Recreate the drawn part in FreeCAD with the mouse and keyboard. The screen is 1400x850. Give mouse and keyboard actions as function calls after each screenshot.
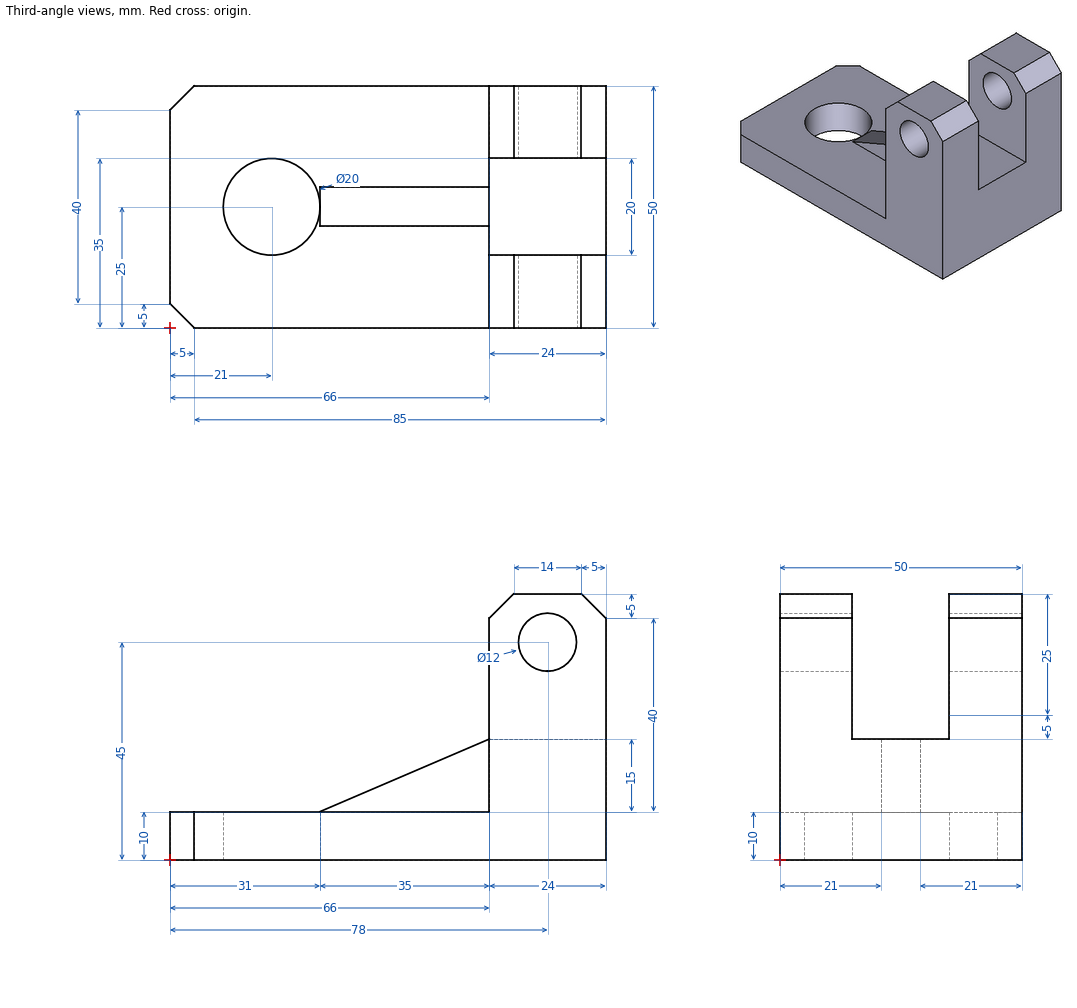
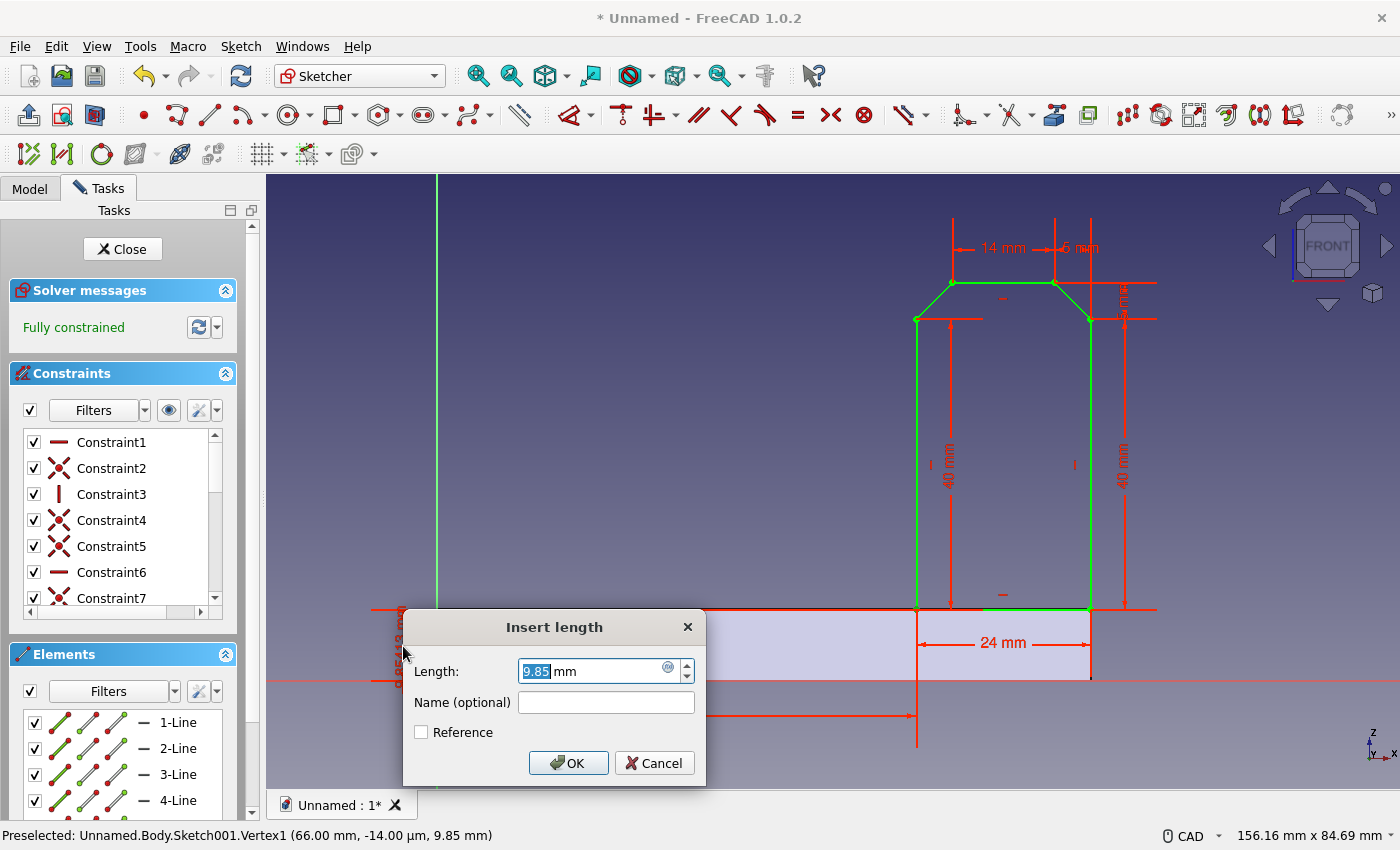
text(10)
key(Return)
key(Escape)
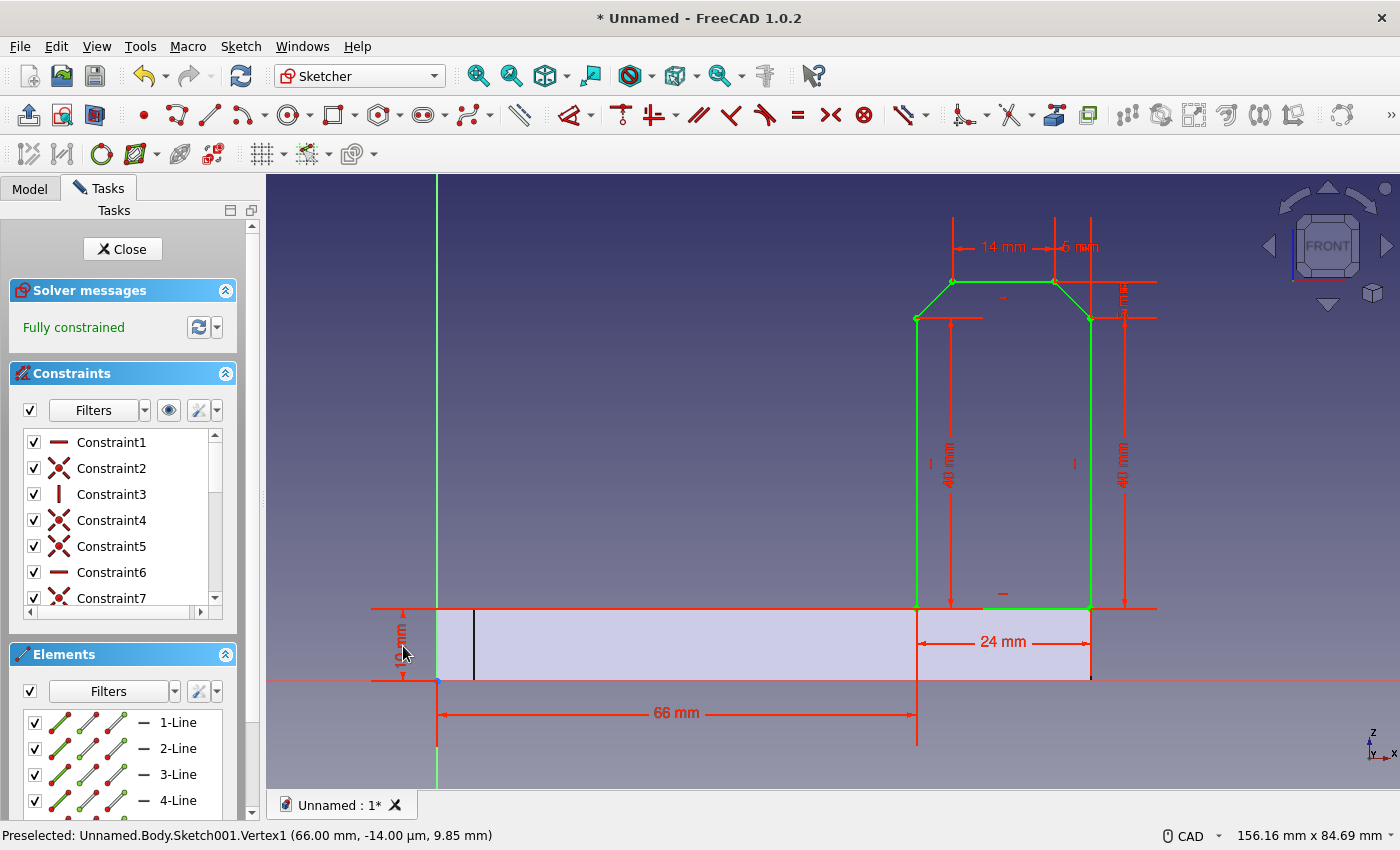
click(123, 249)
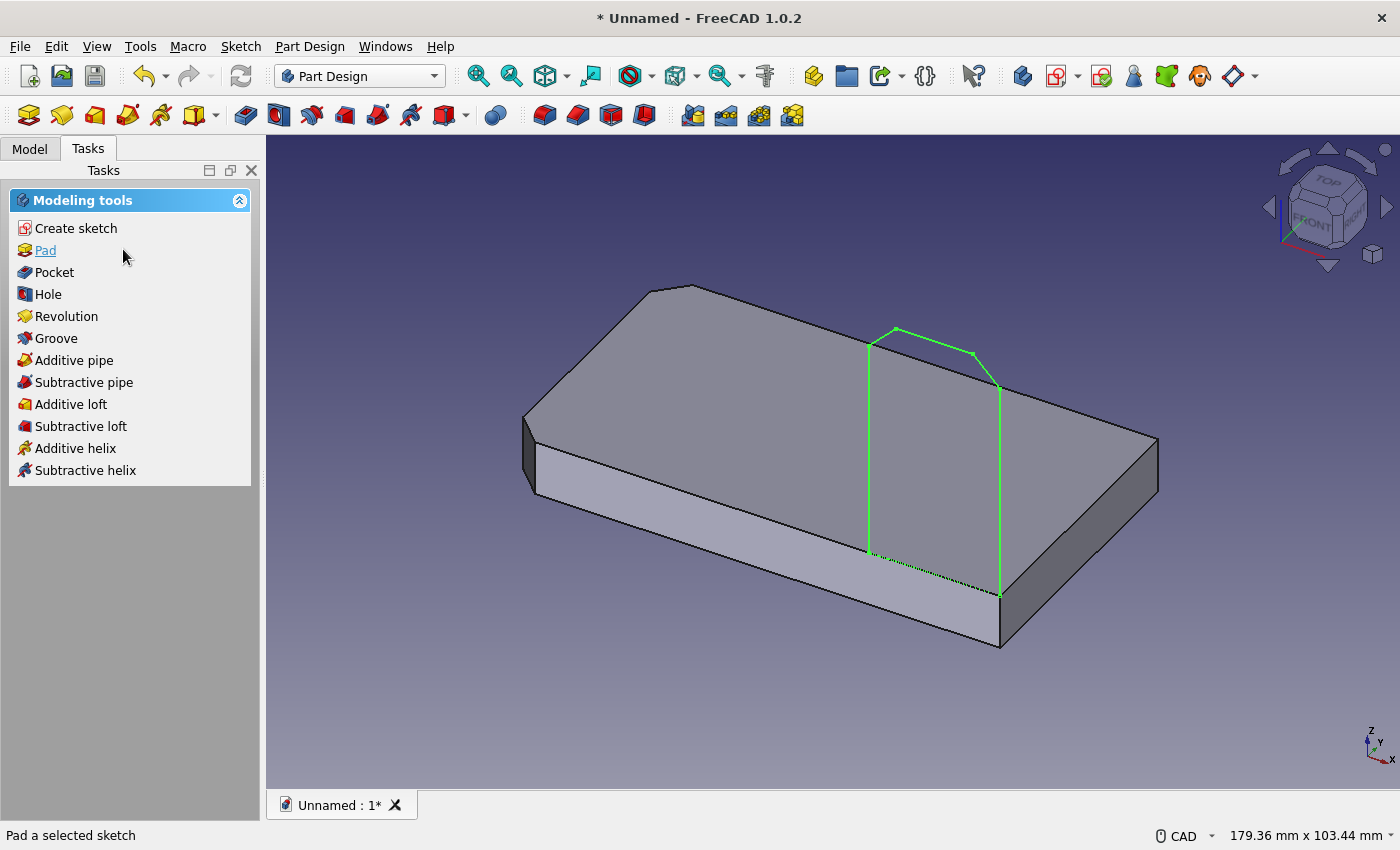
click(29, 116)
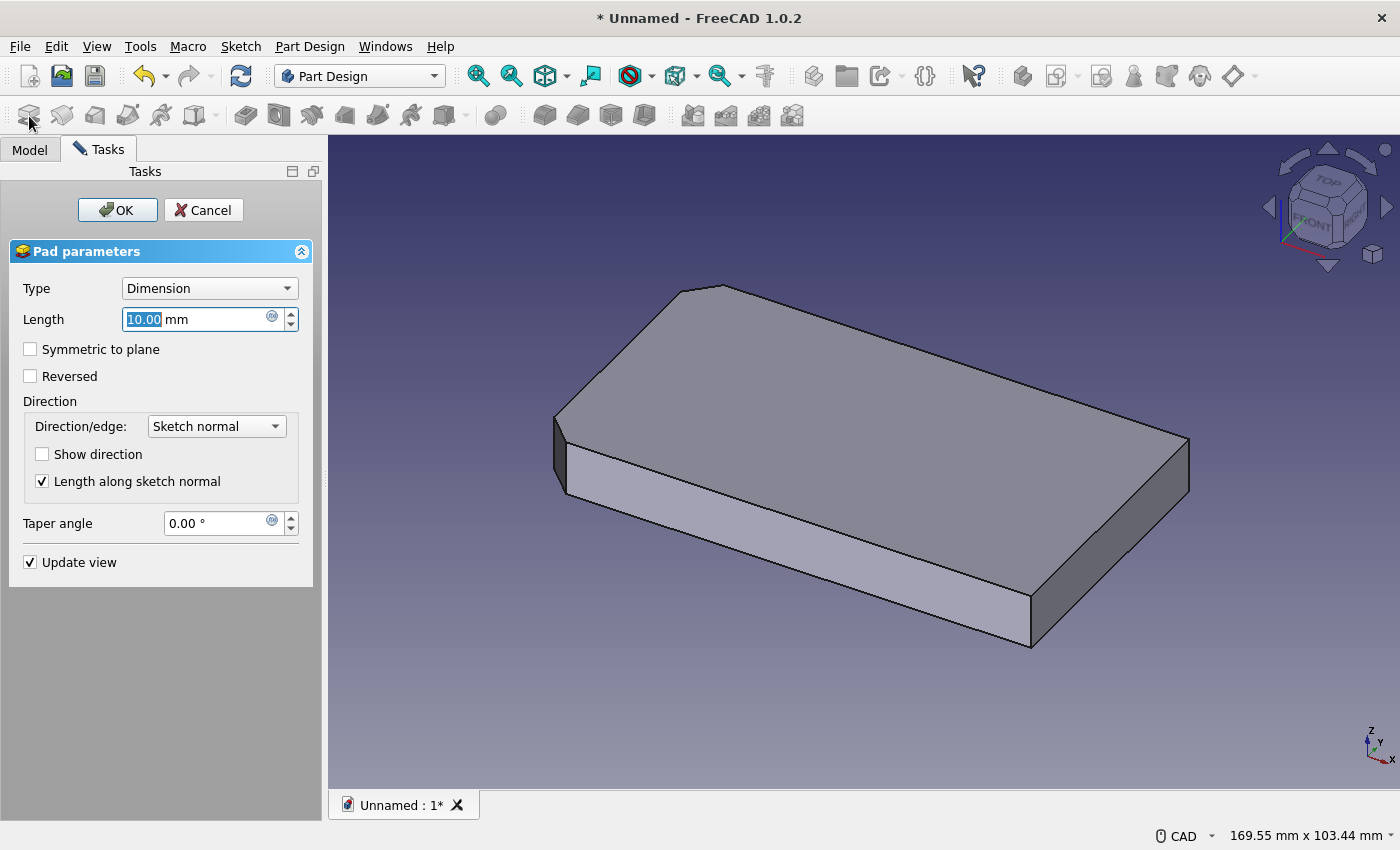
text(50)
key(Tab)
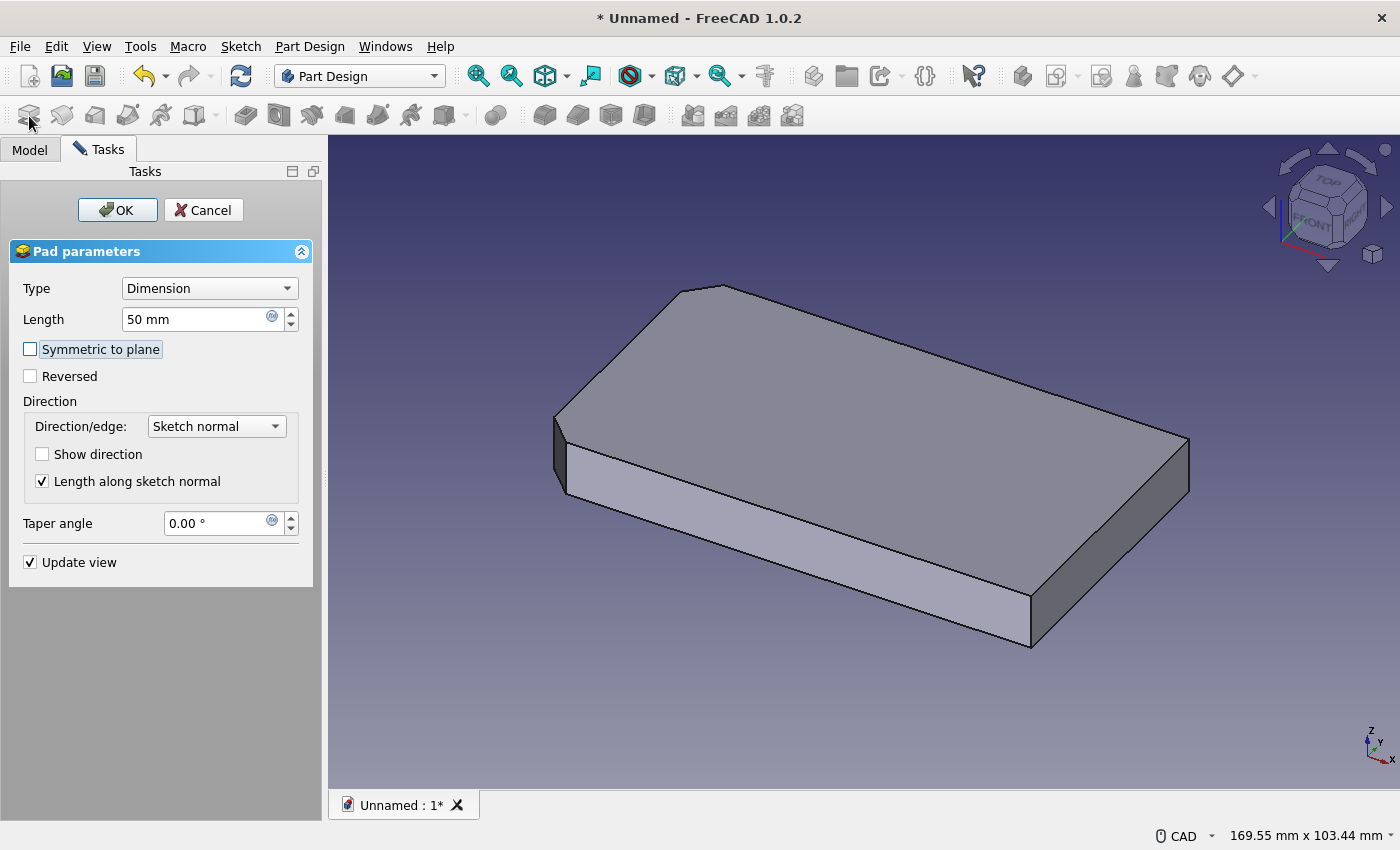
click(31, 376)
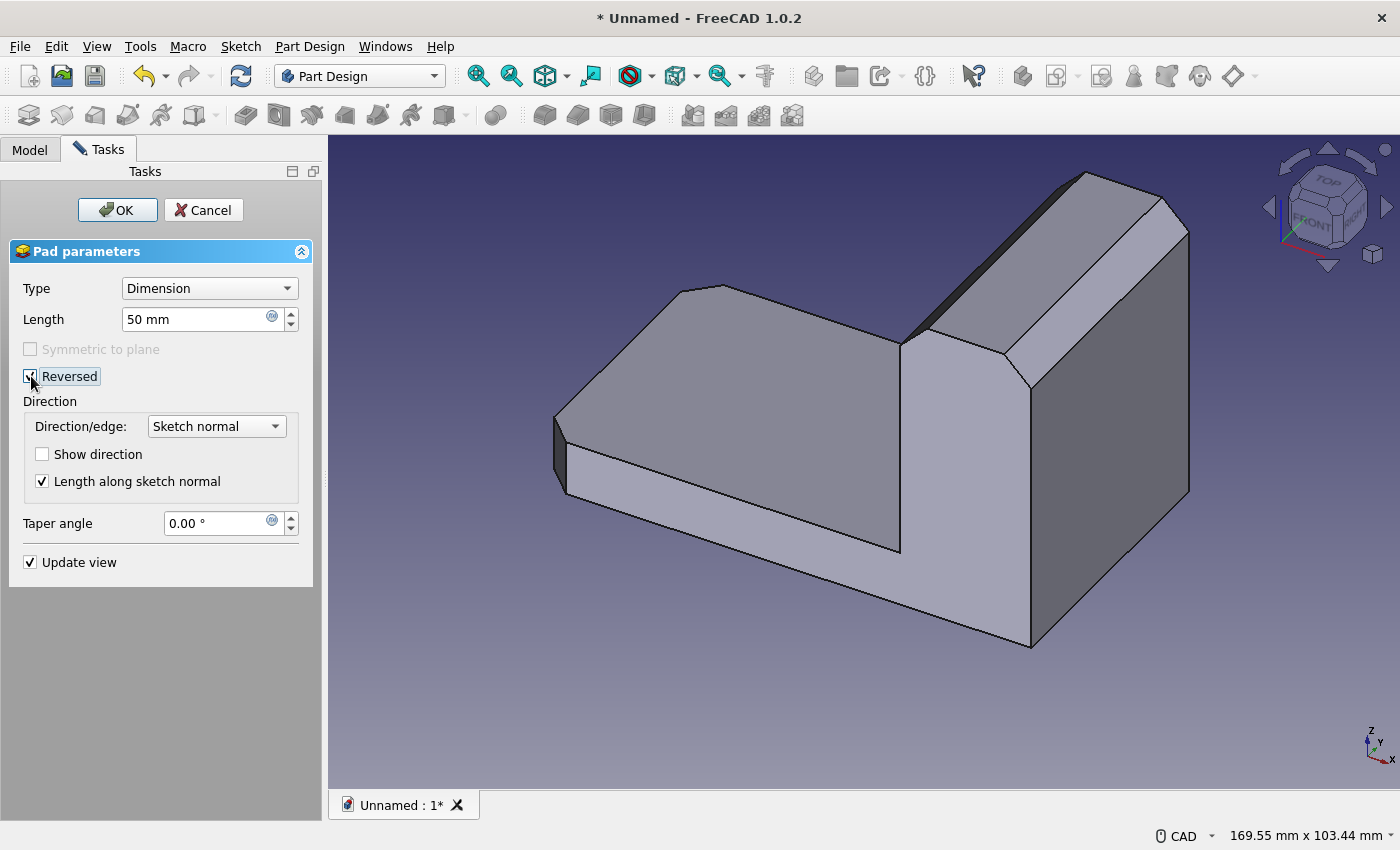
click(118, 210)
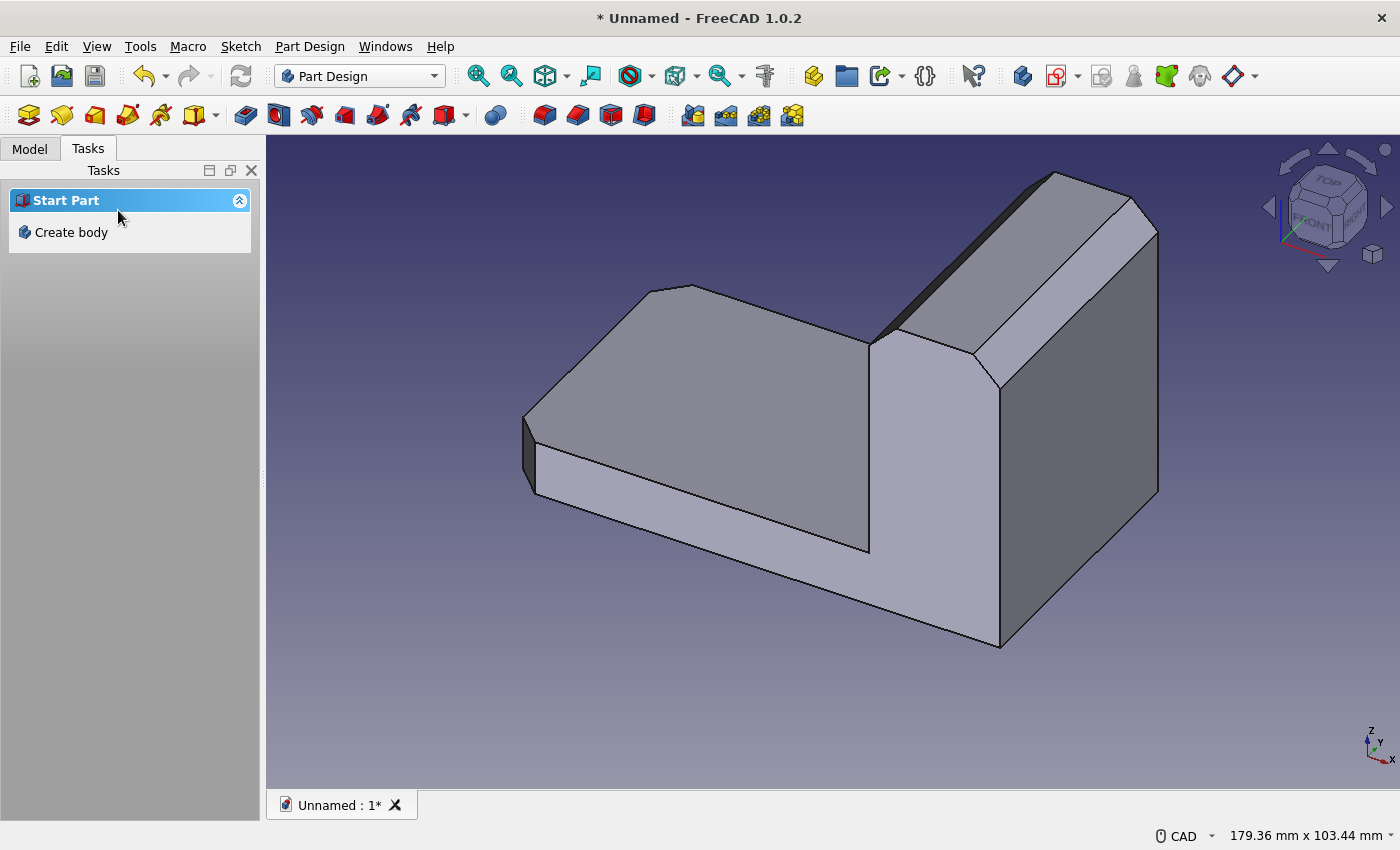
click(479, 76)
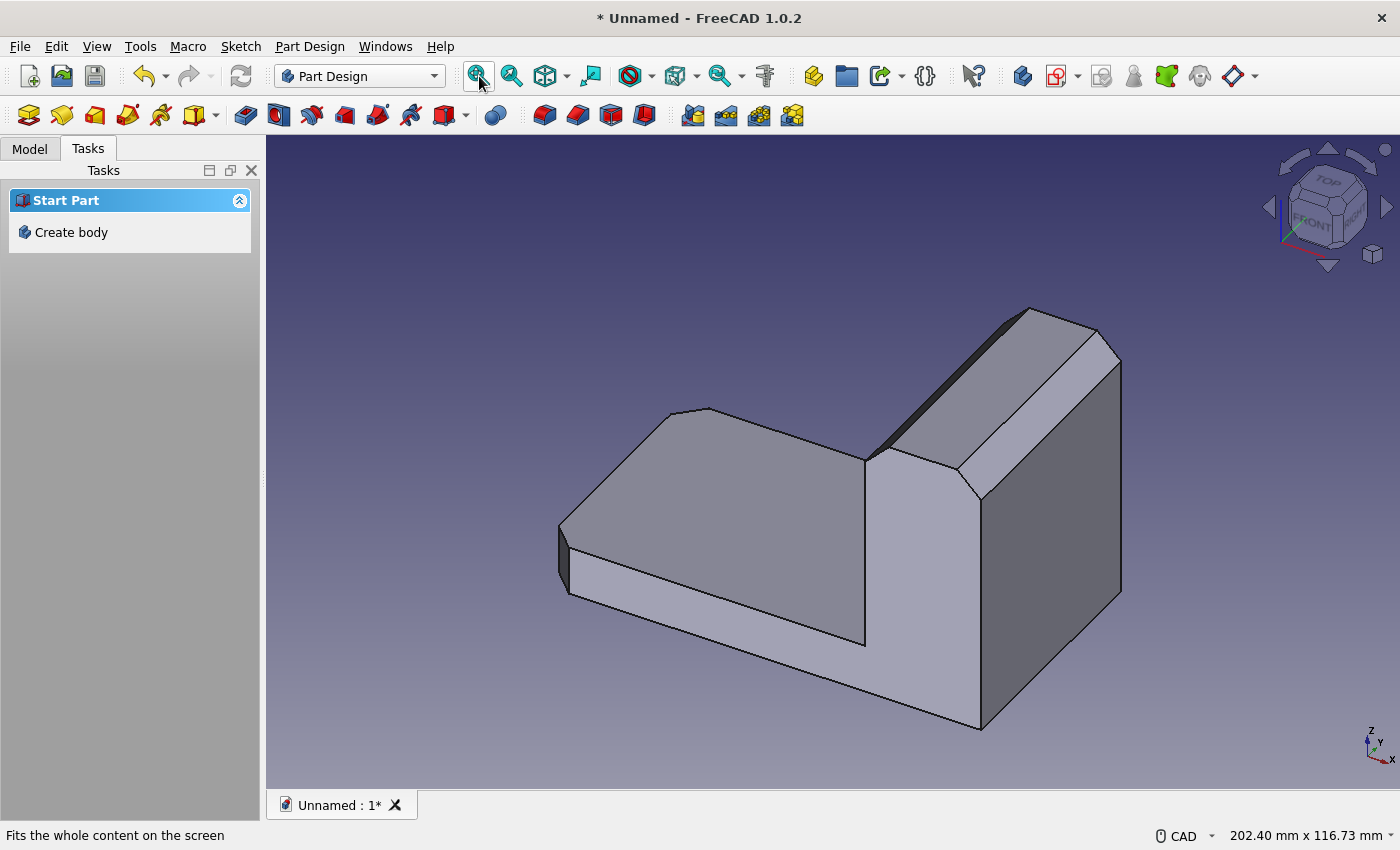
click(1056, 76)